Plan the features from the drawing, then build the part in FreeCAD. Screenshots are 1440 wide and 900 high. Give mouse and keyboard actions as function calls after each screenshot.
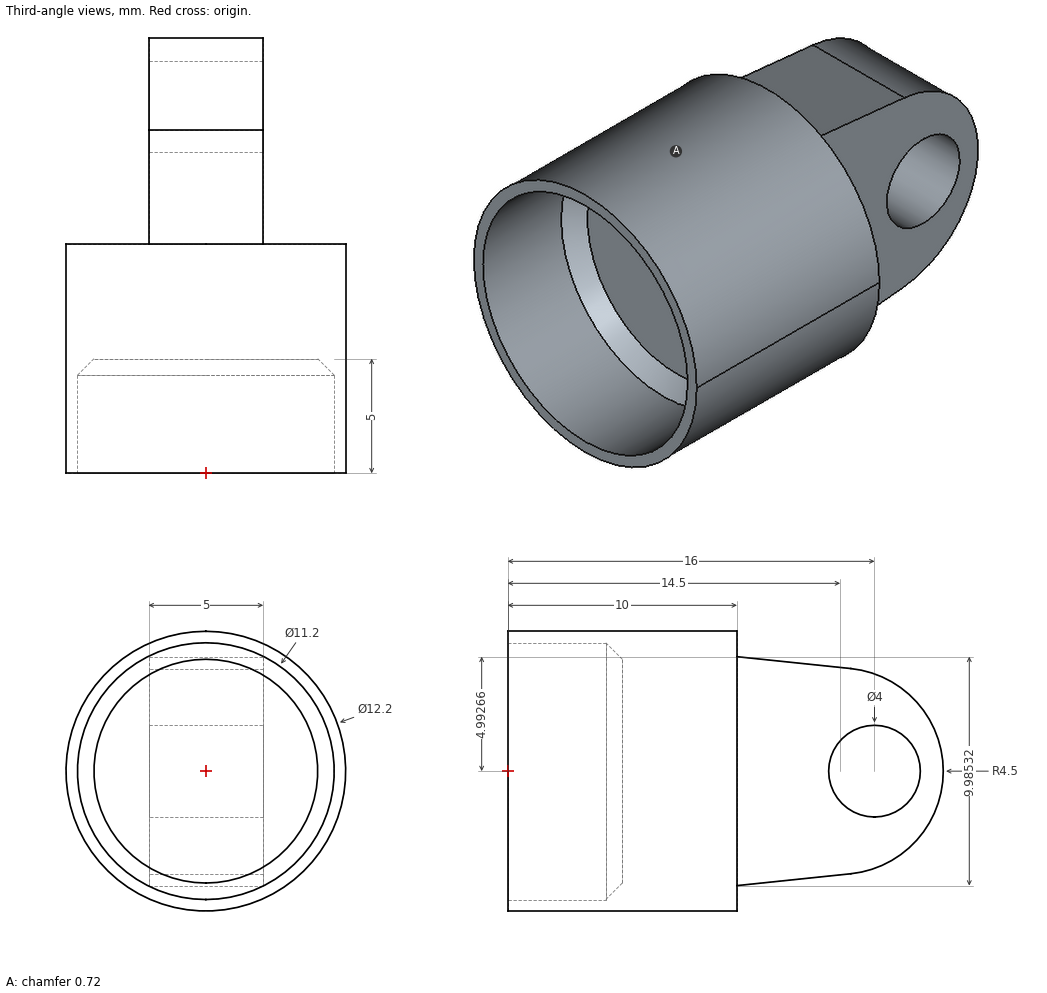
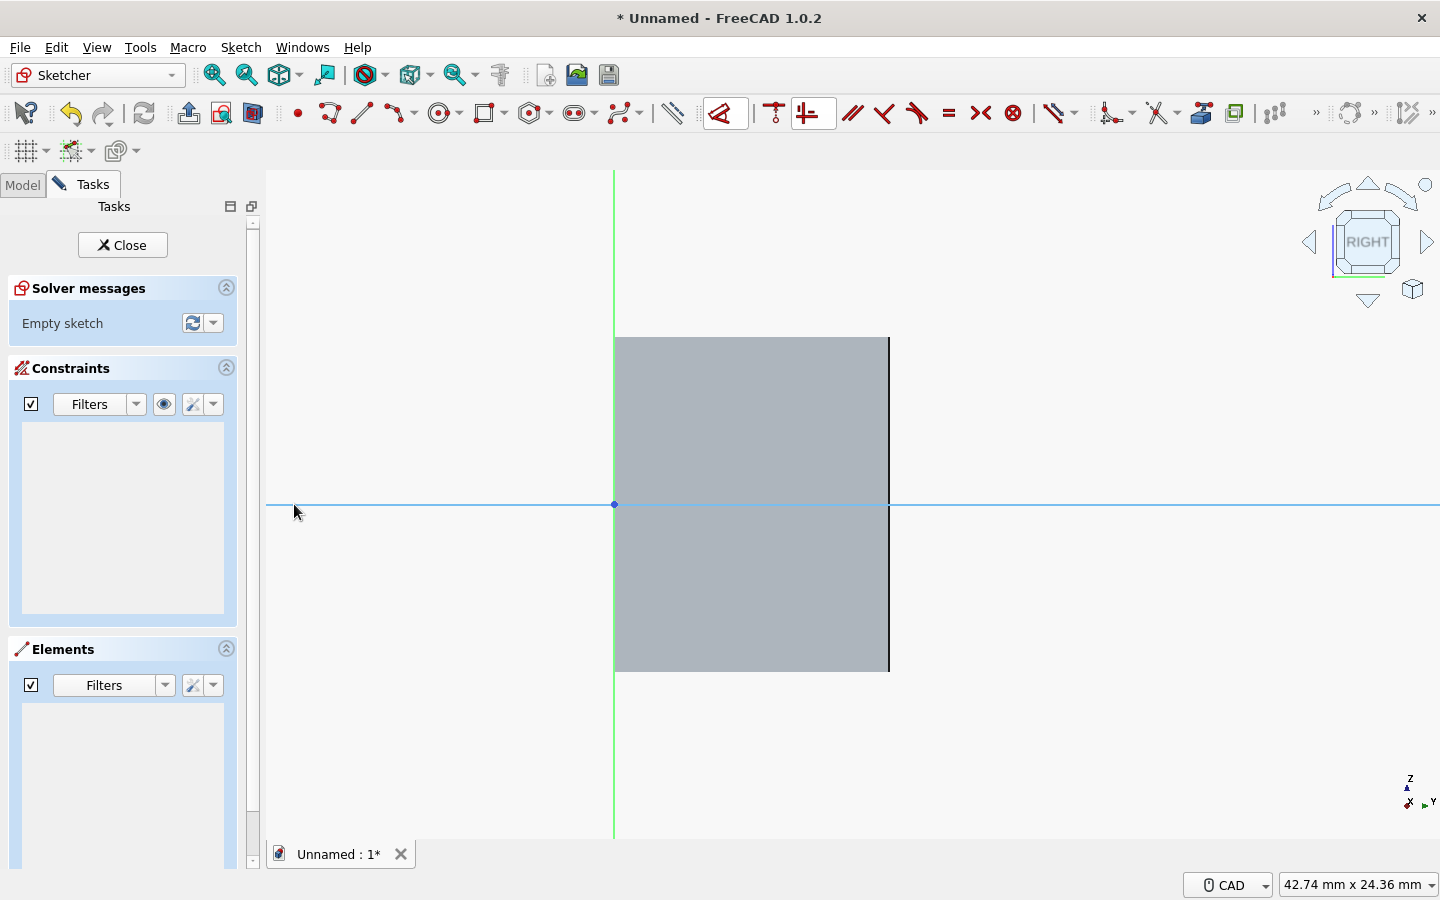
key(g)
key(m)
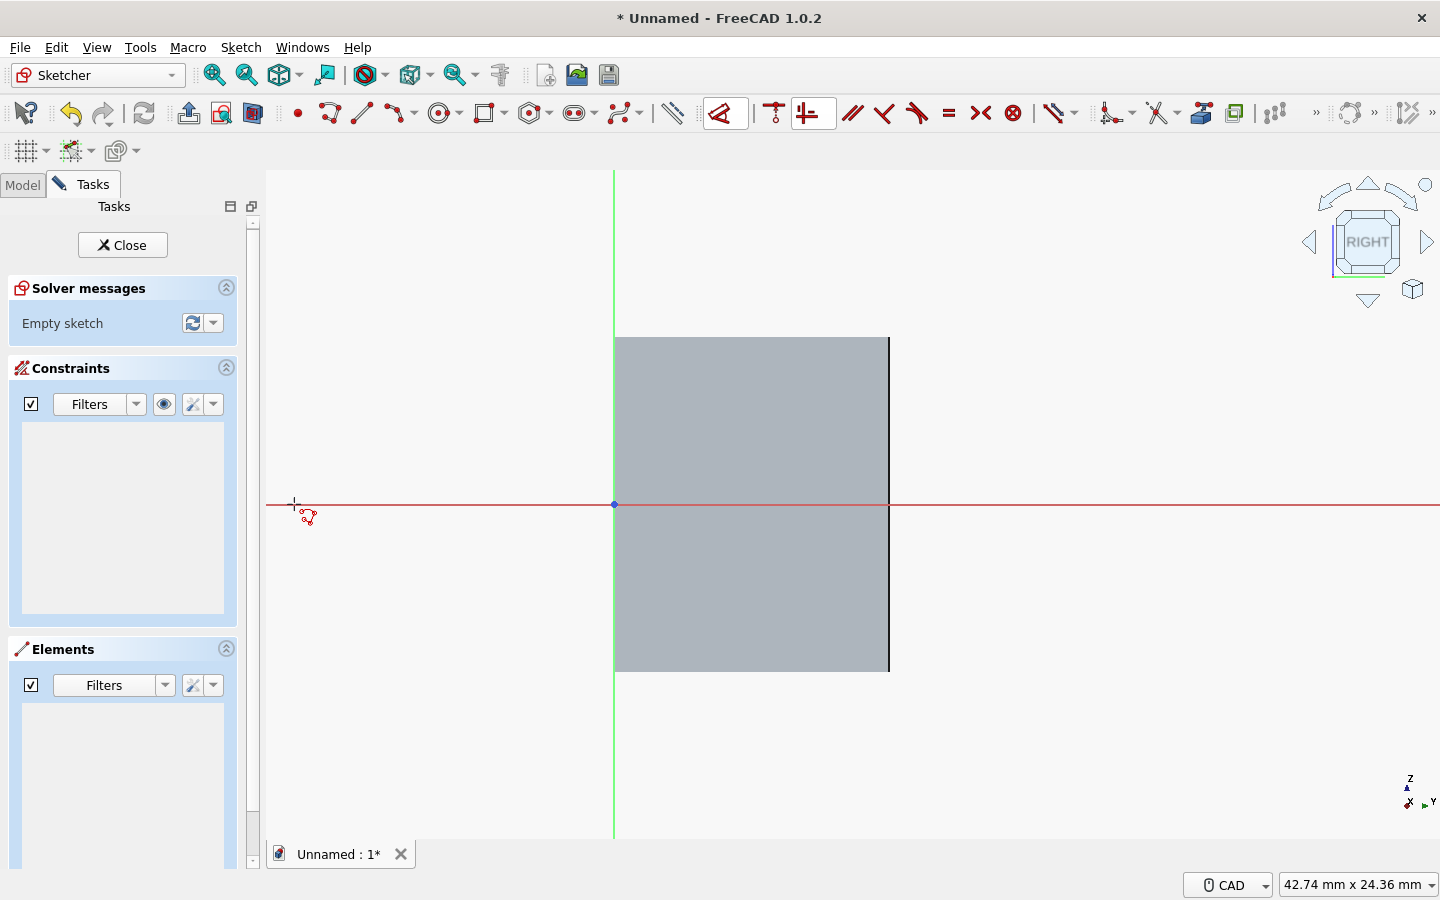
click(1025, 382)
click(889, 367)
click(889, 642)
click(1025, 627)
right_click(1025, 627)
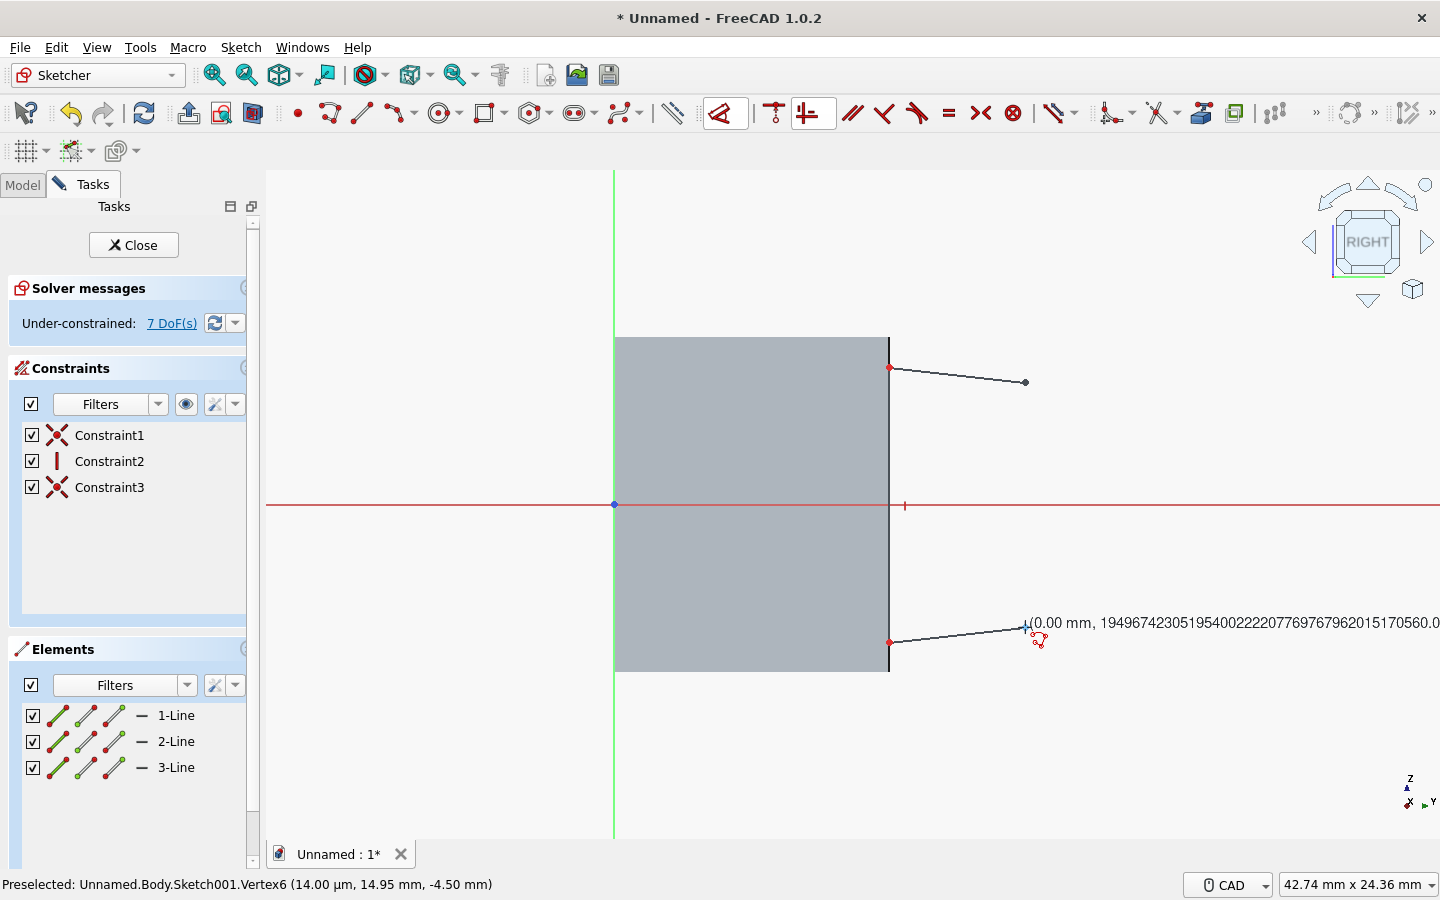
click(394, 114)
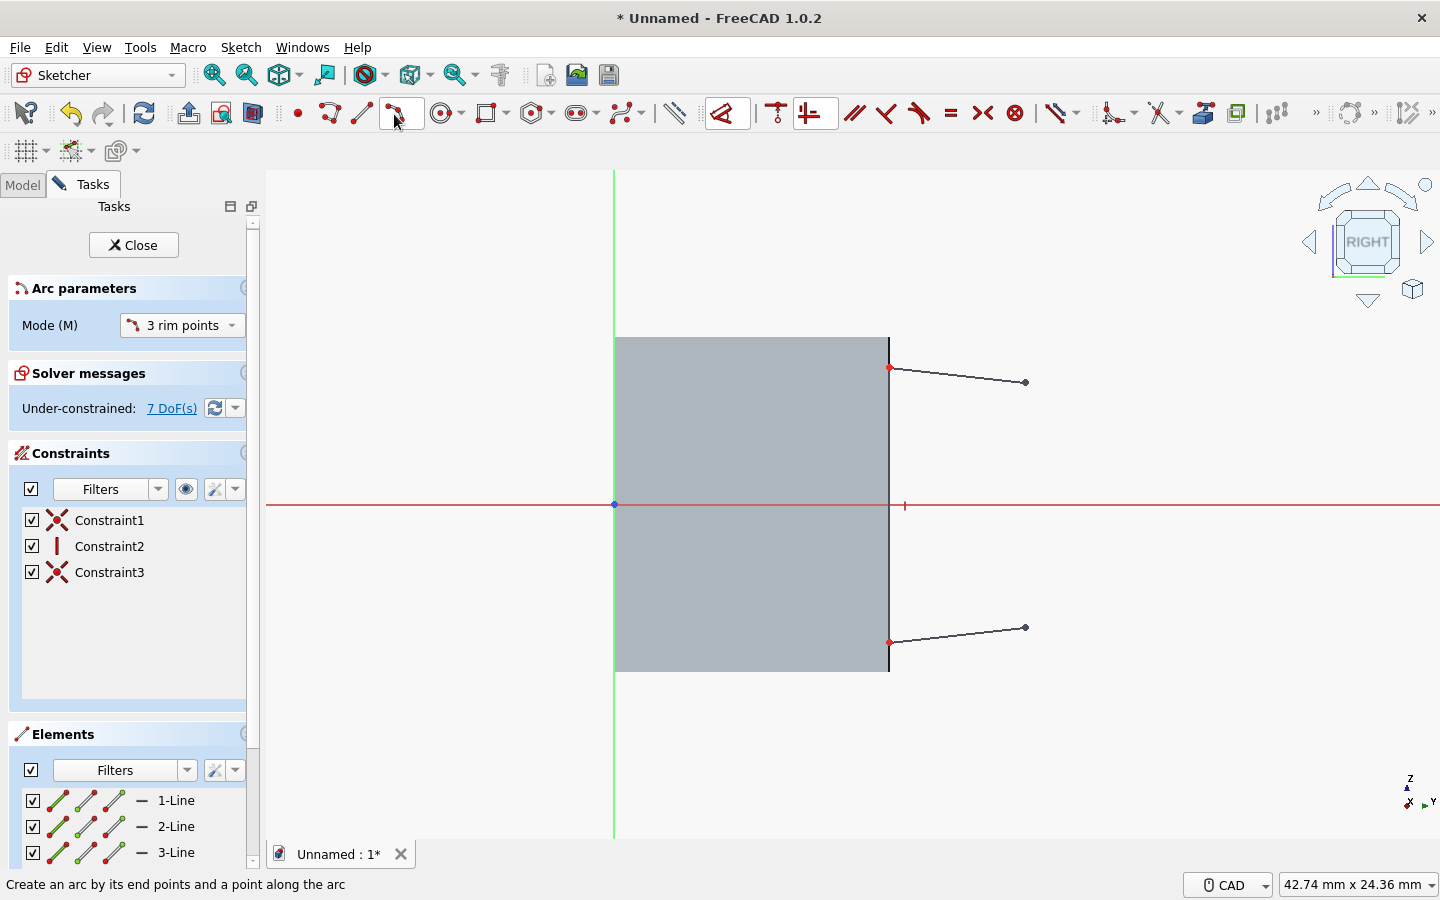
click(1025, 628)
click(1025, 383)
click(1131, 540)
key(Escape)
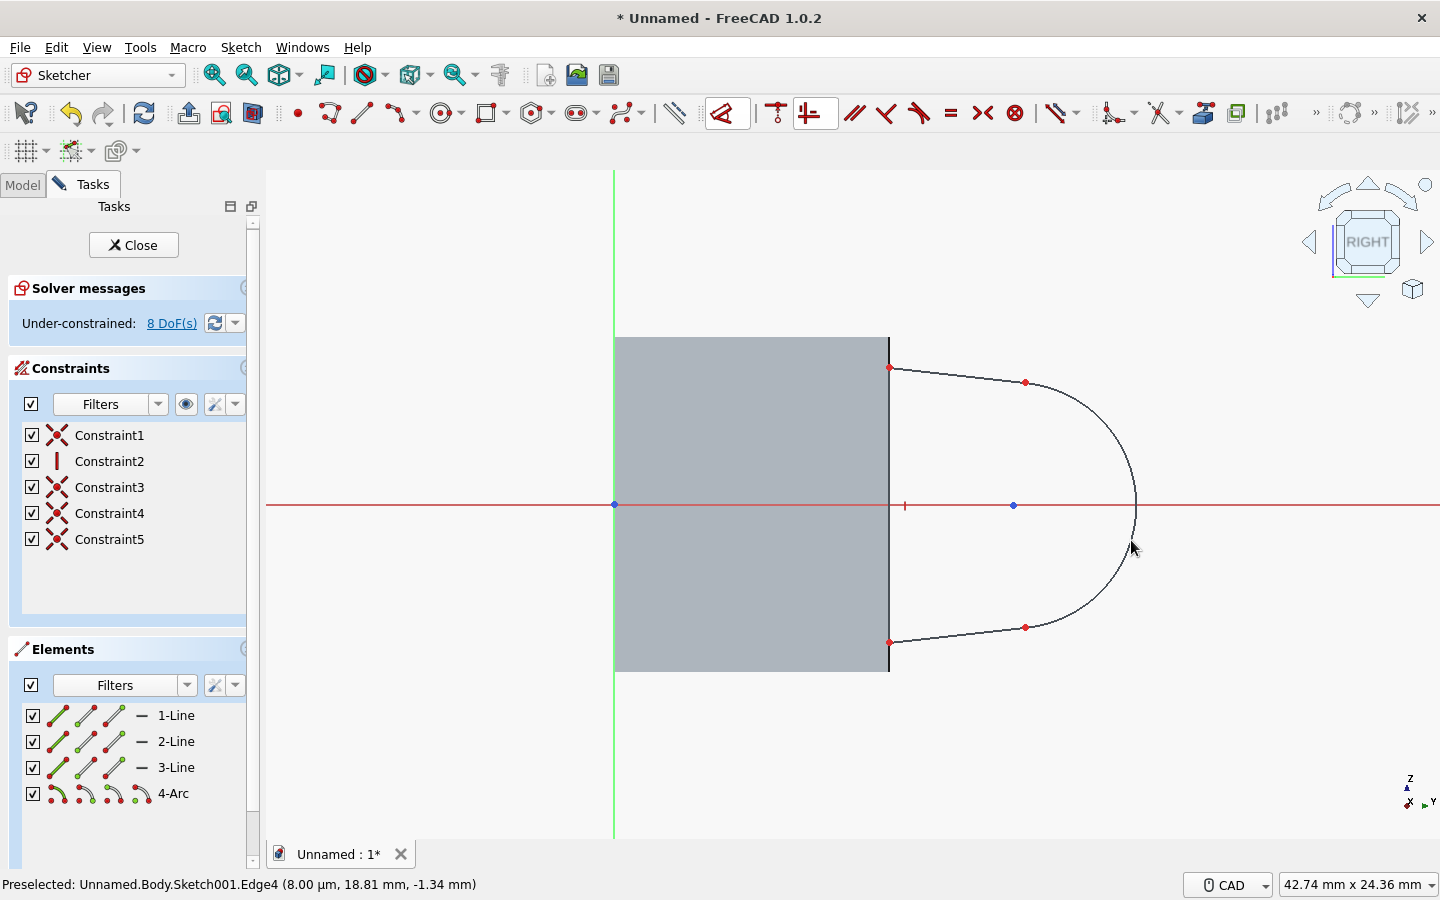
click(984, 378)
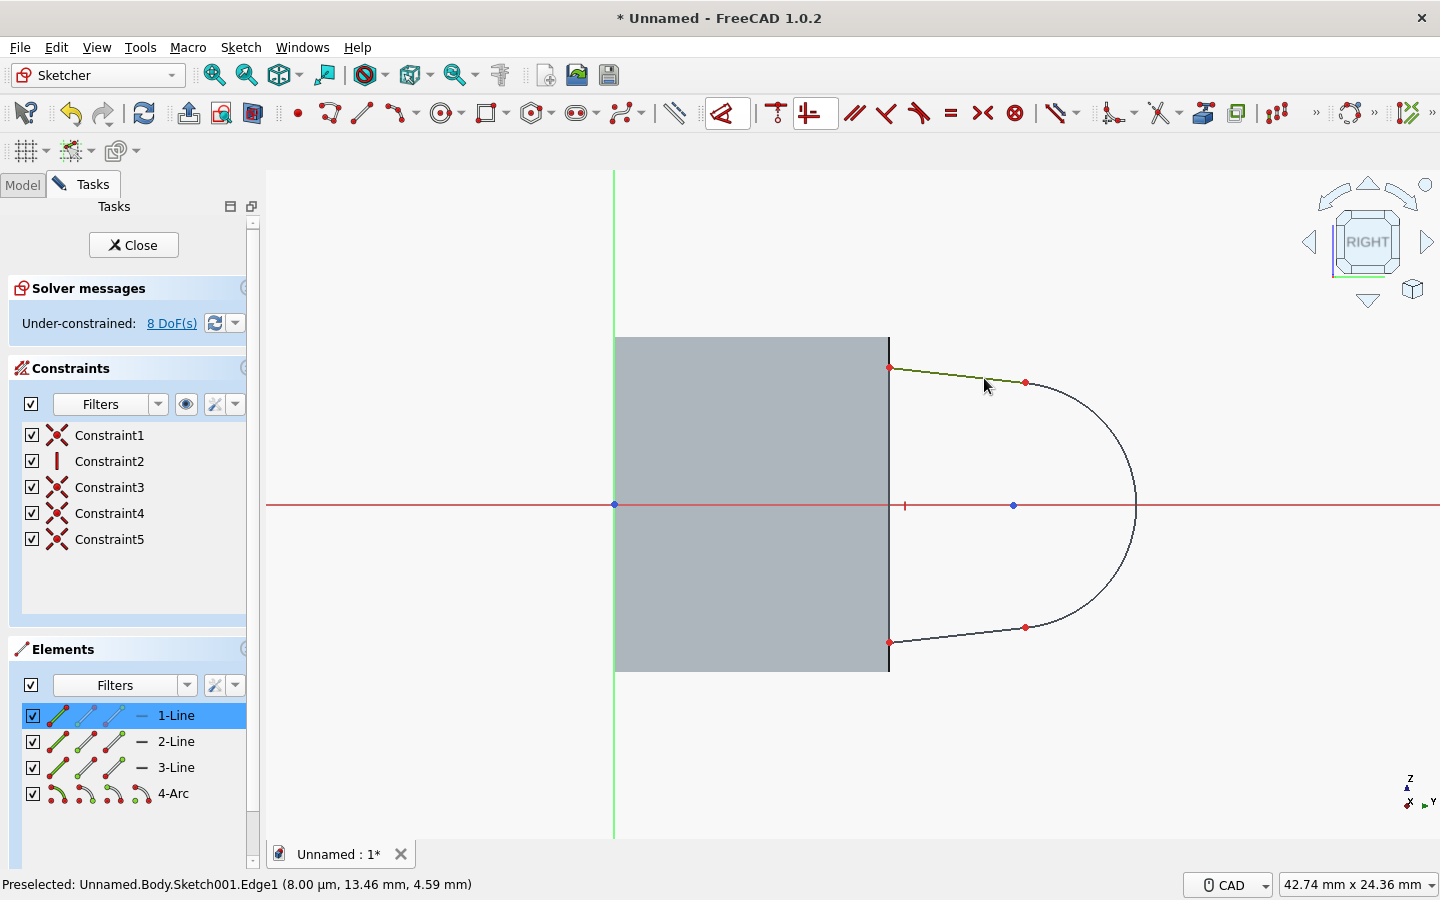
click(1115, 574)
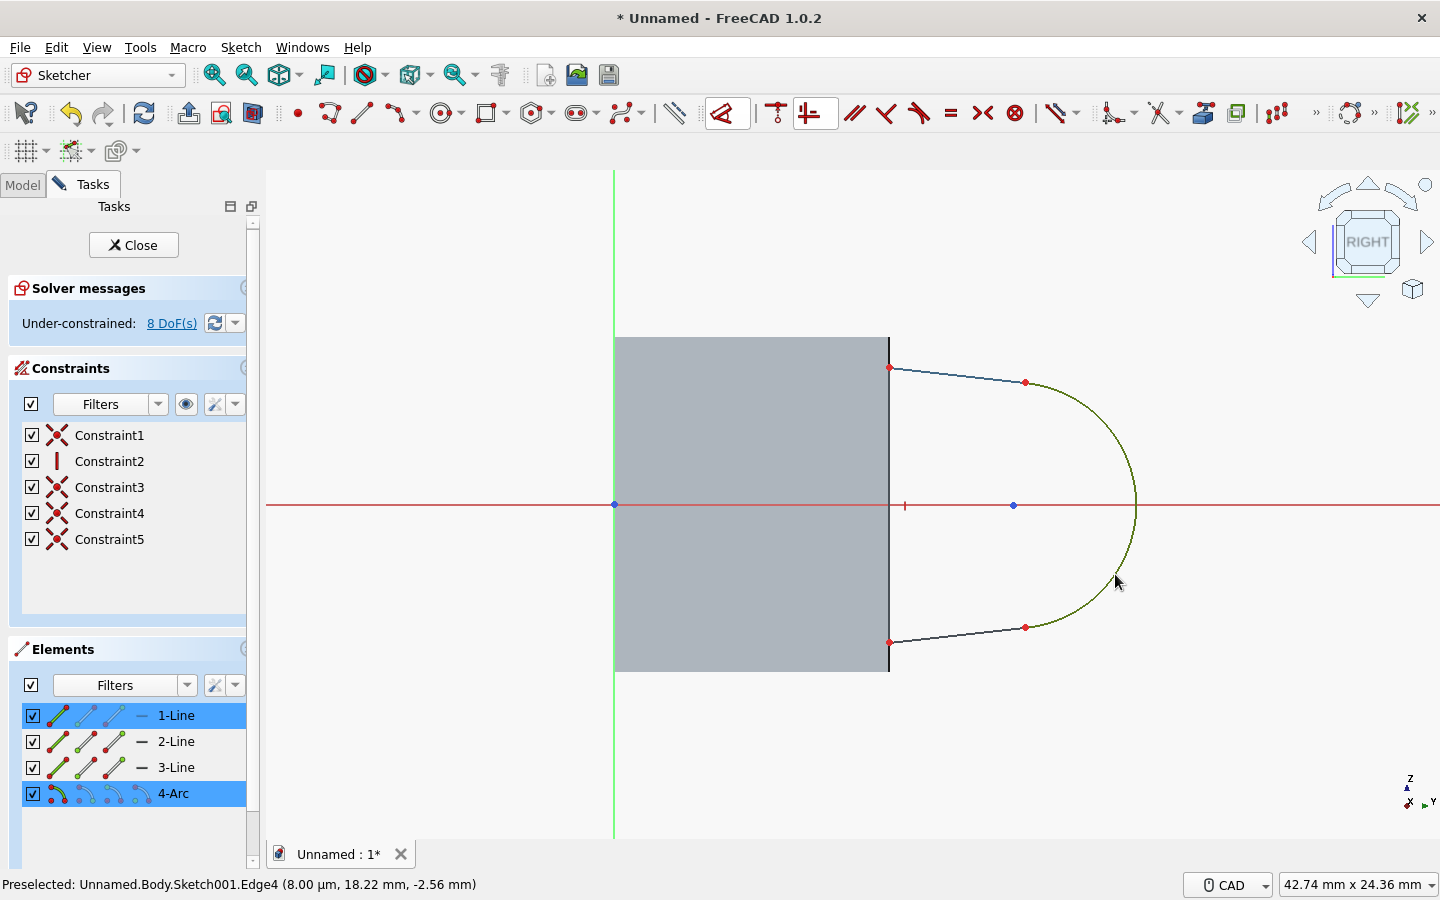
click(920, 114)